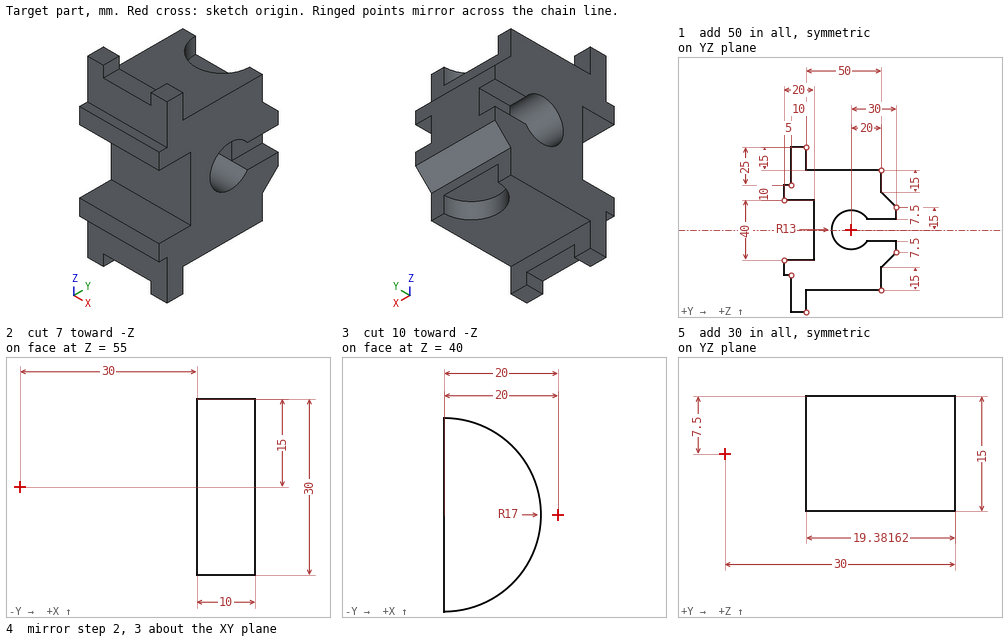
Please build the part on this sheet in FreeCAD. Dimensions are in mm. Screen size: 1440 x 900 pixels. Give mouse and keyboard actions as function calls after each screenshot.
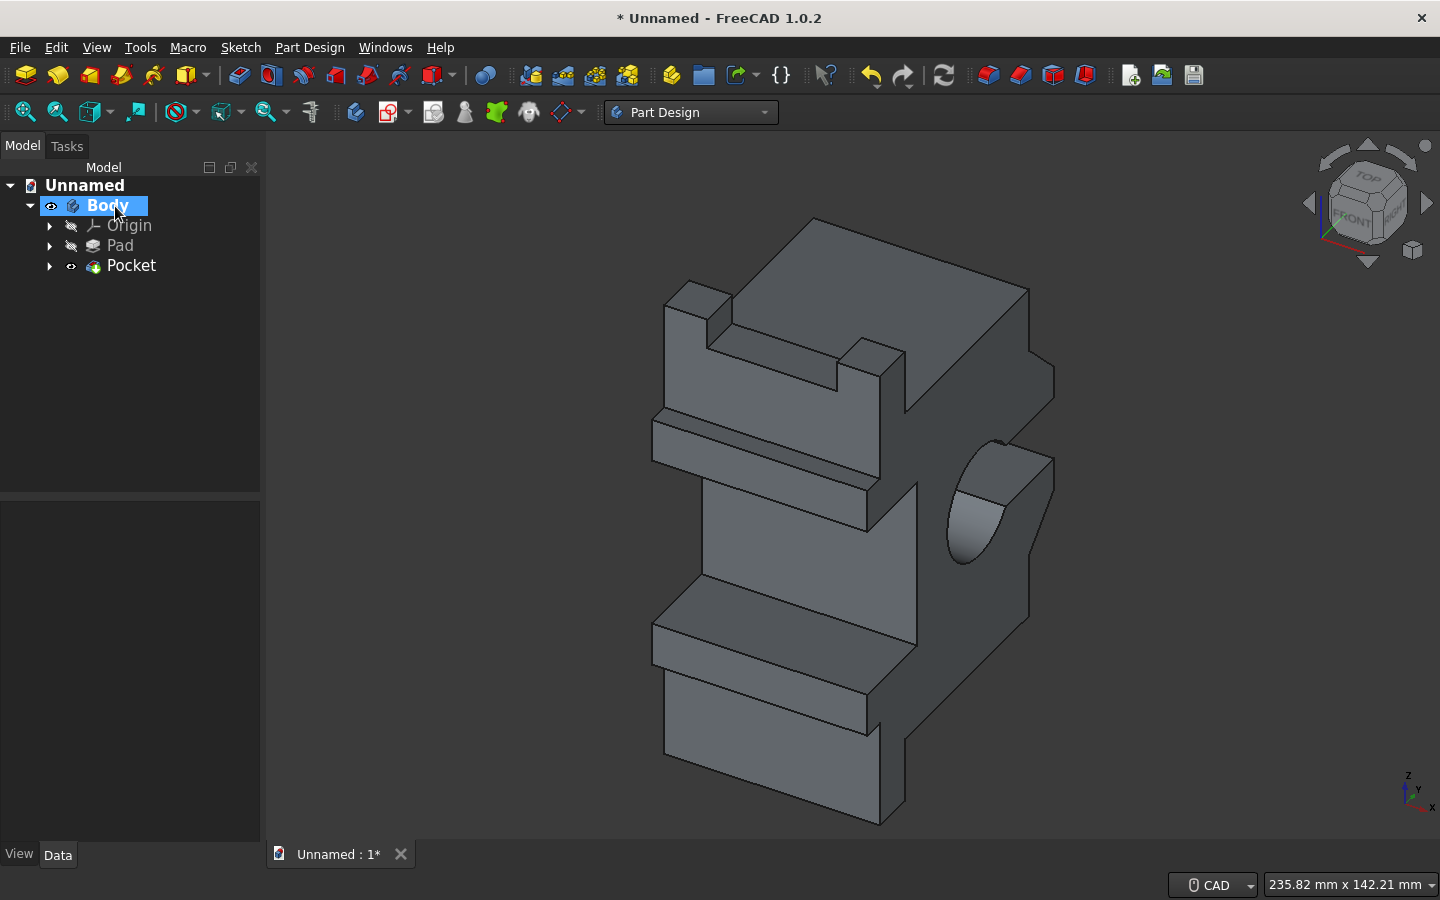
click(859, 315)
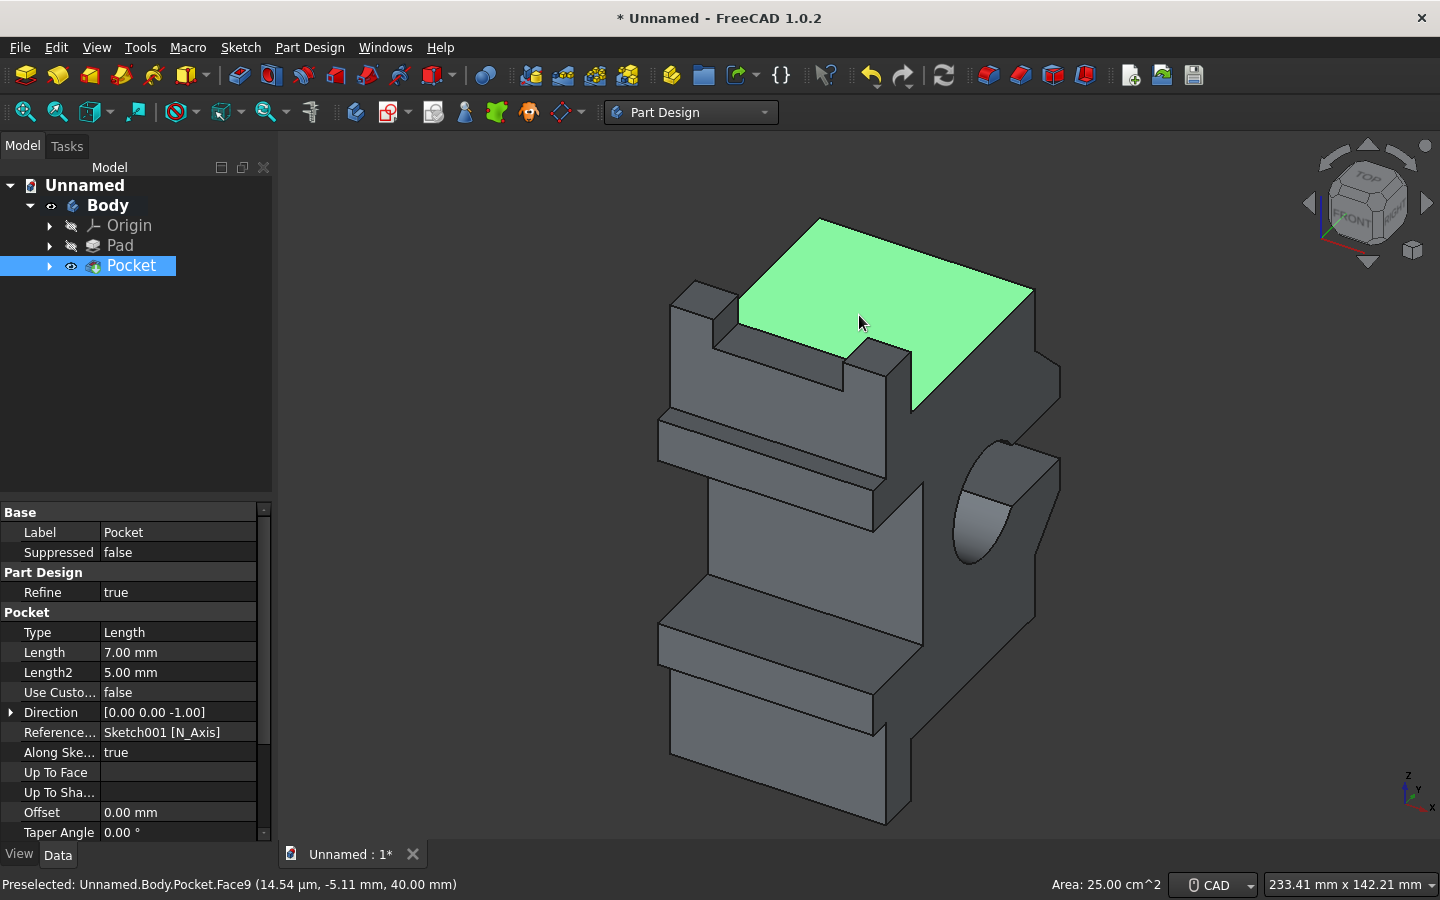
click(388, 112)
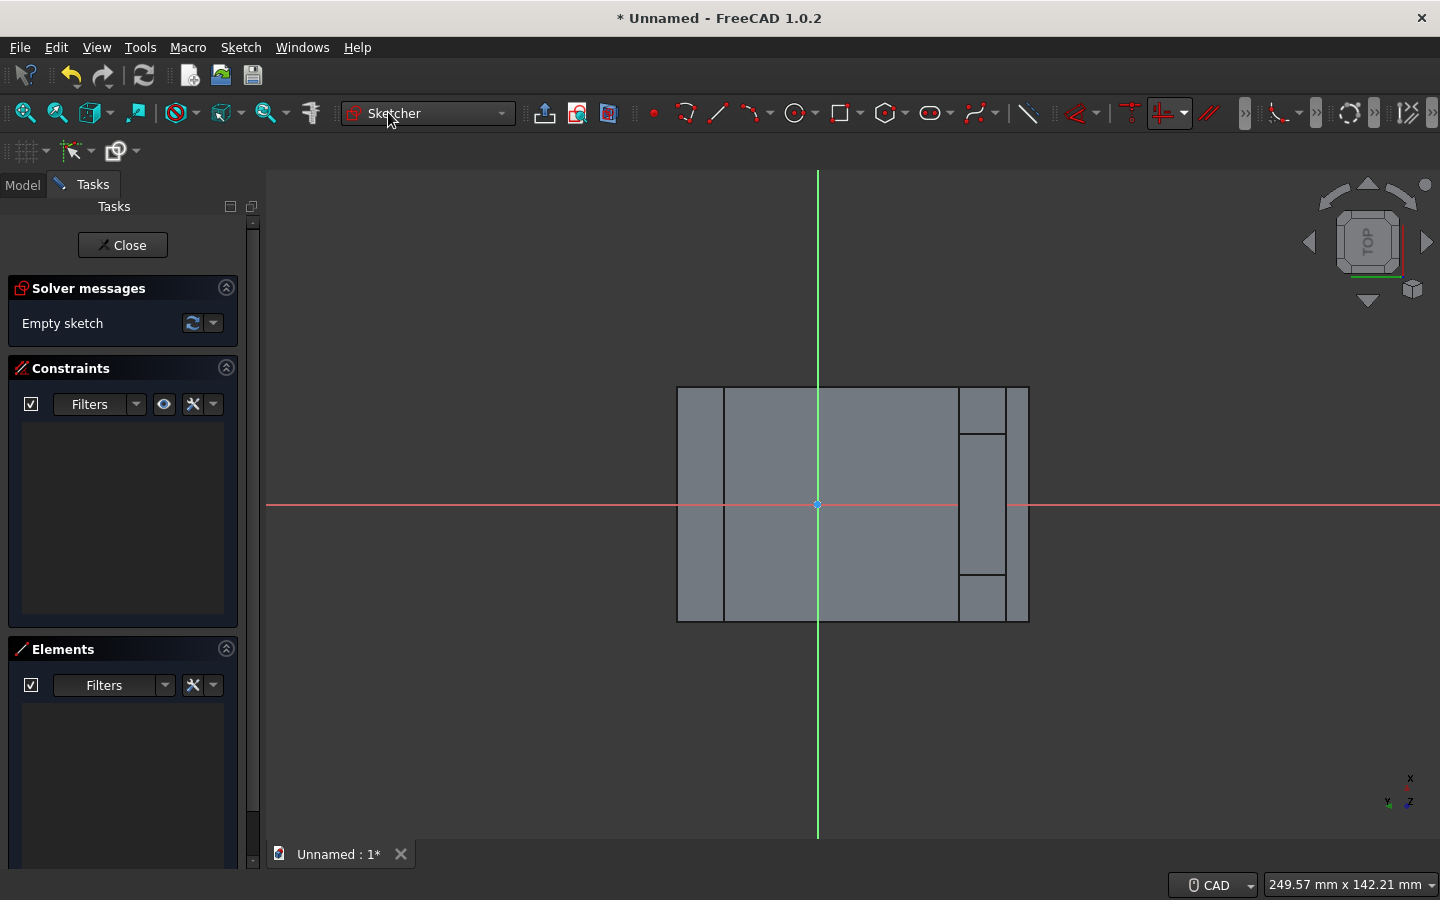
scroll(763, 504, up, 5)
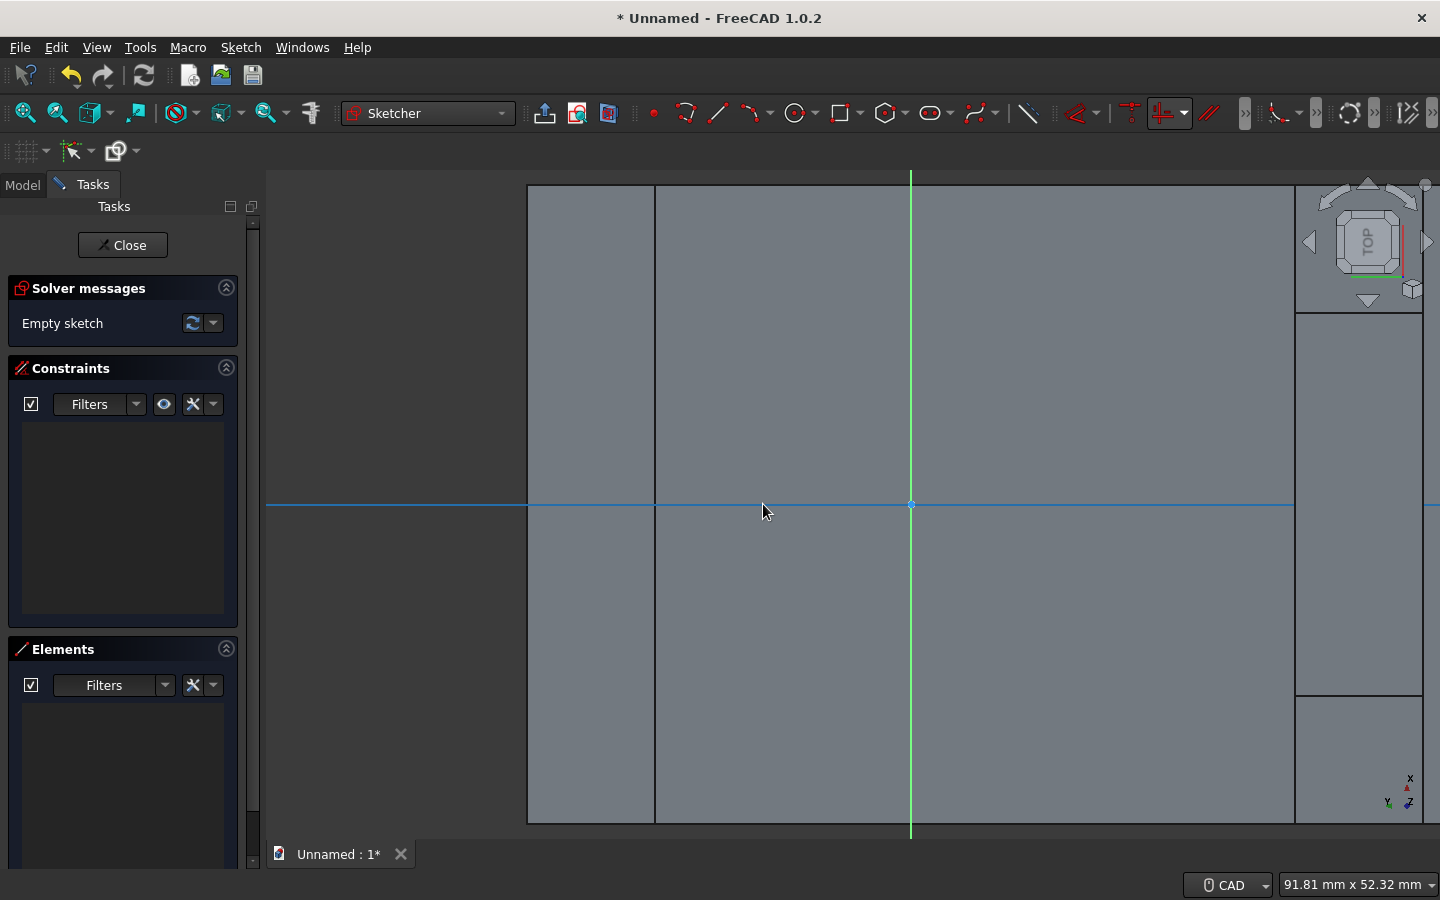
click(718, 114)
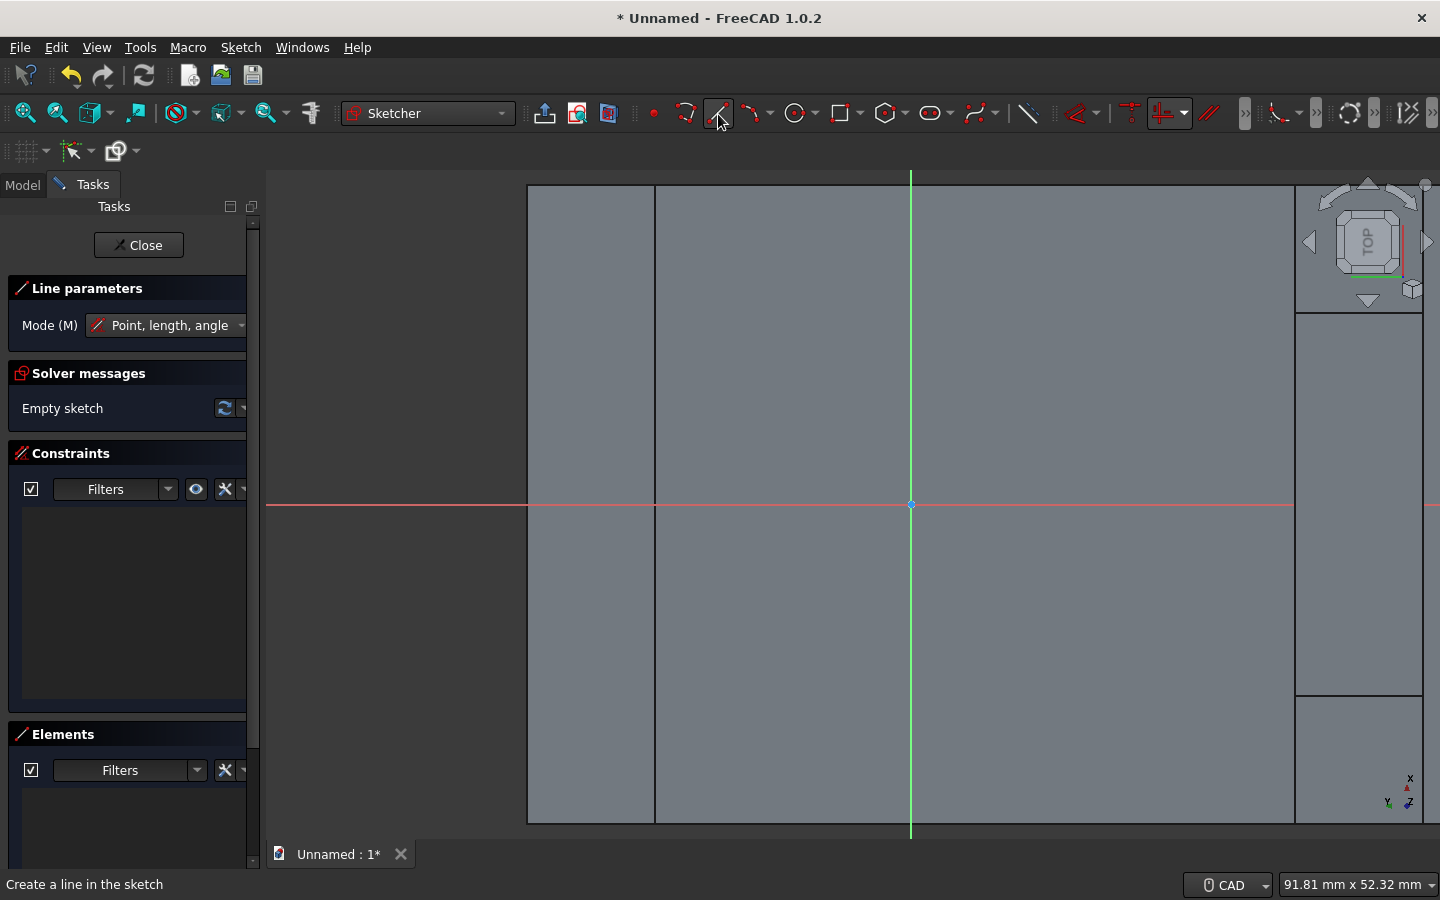
click(655, 287)
click(655, 722)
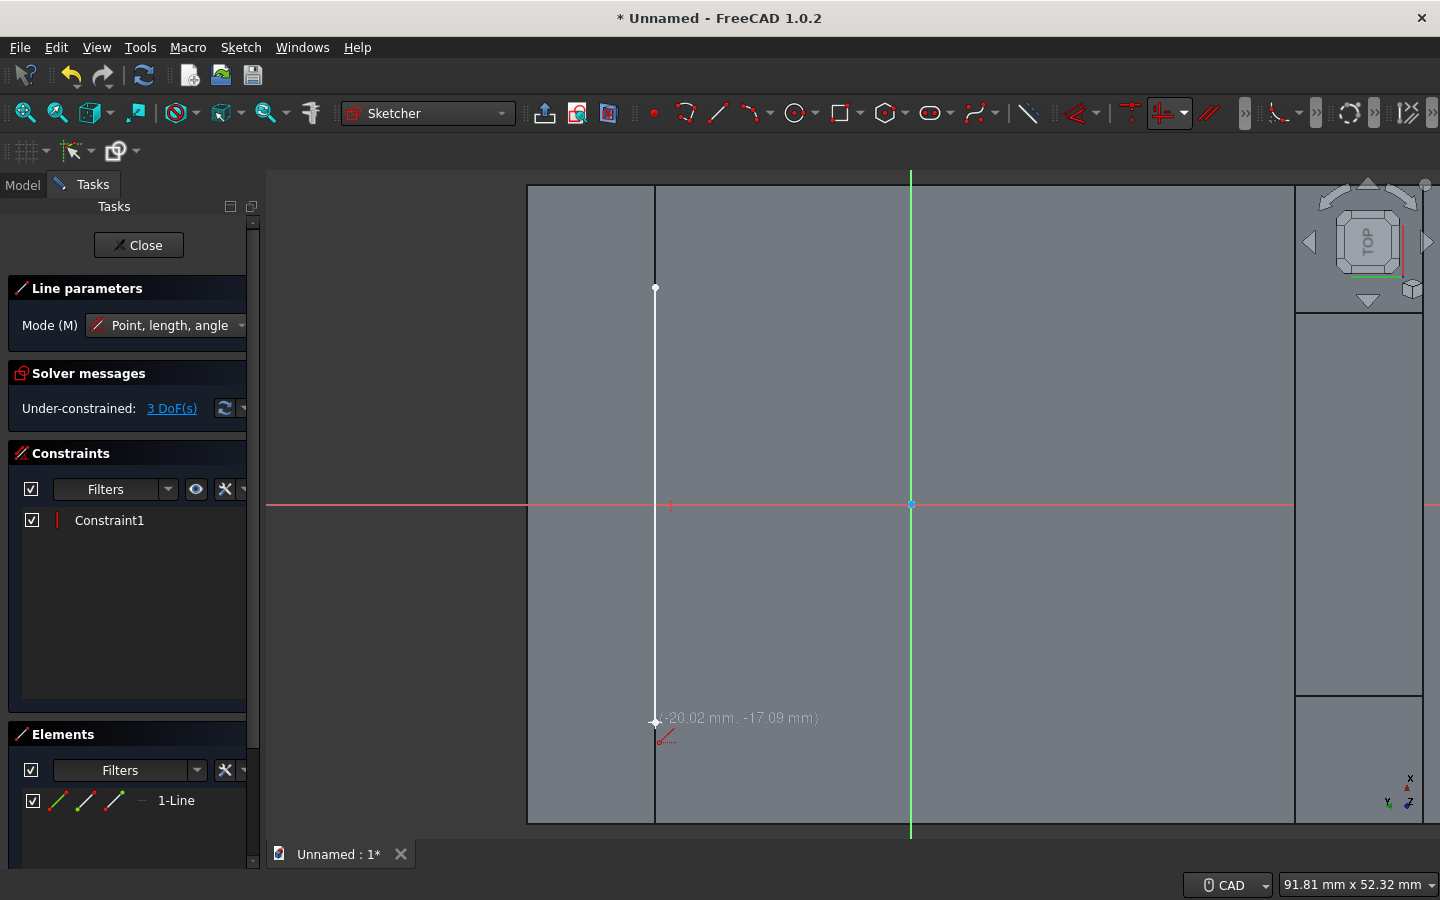
click(750, 114)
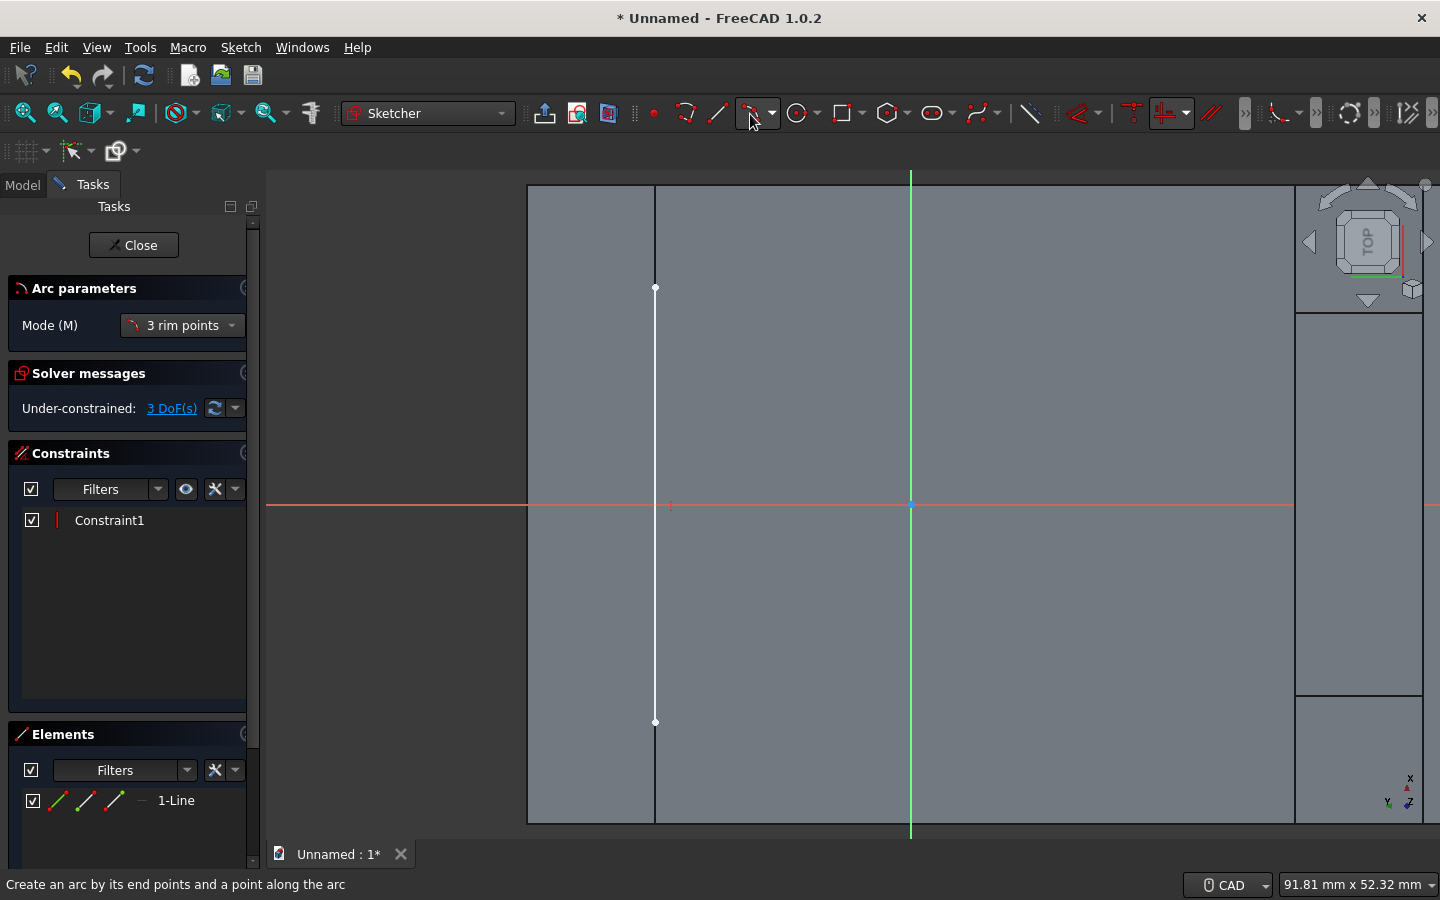
click(655, 723)
click(655, 288)
click(862, 572)
key(Escape)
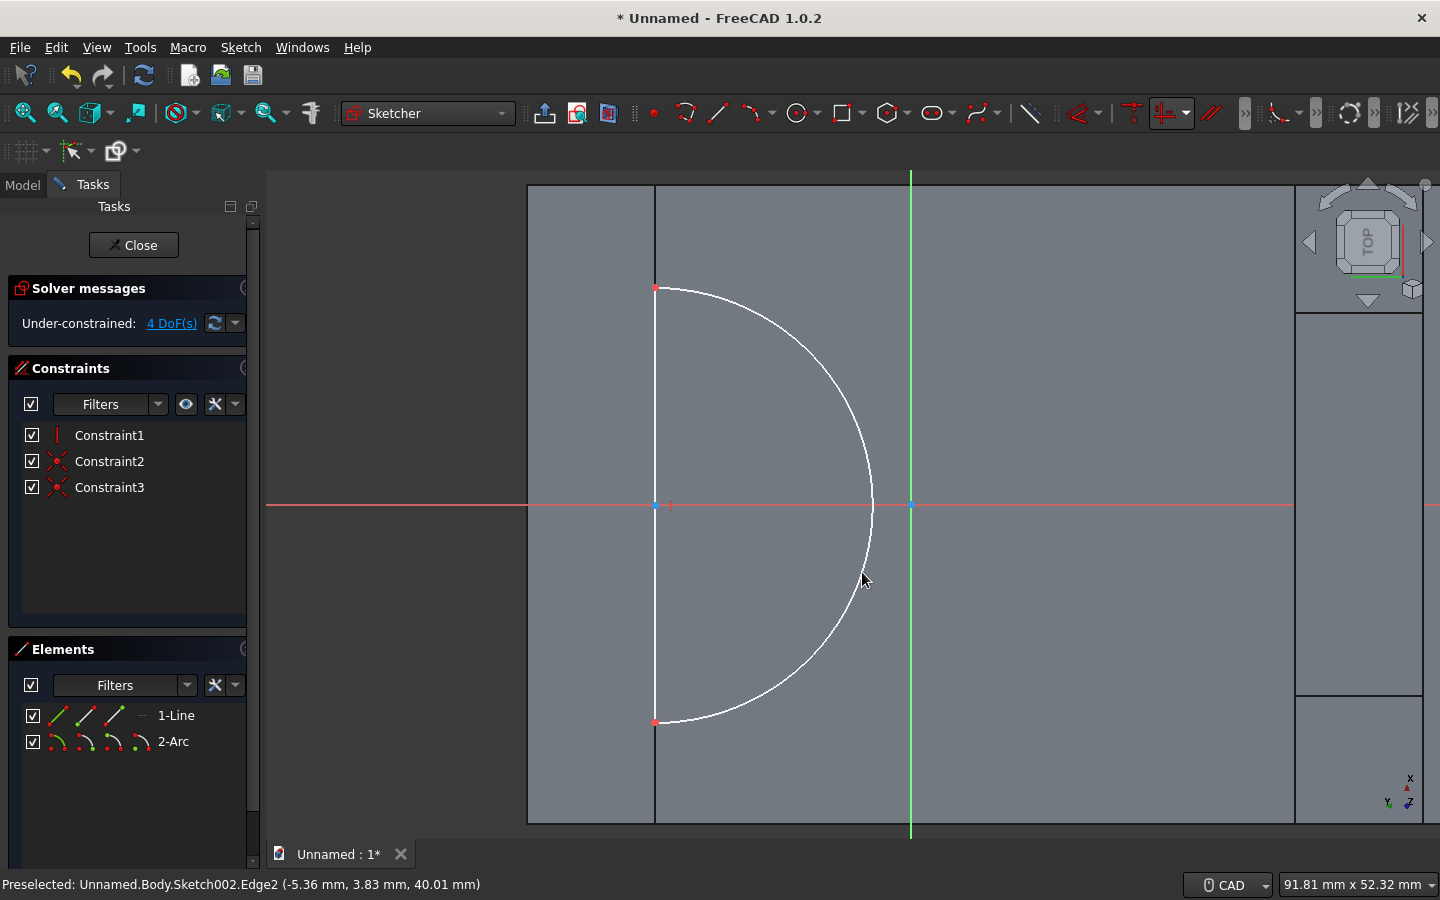
click(655, 506)